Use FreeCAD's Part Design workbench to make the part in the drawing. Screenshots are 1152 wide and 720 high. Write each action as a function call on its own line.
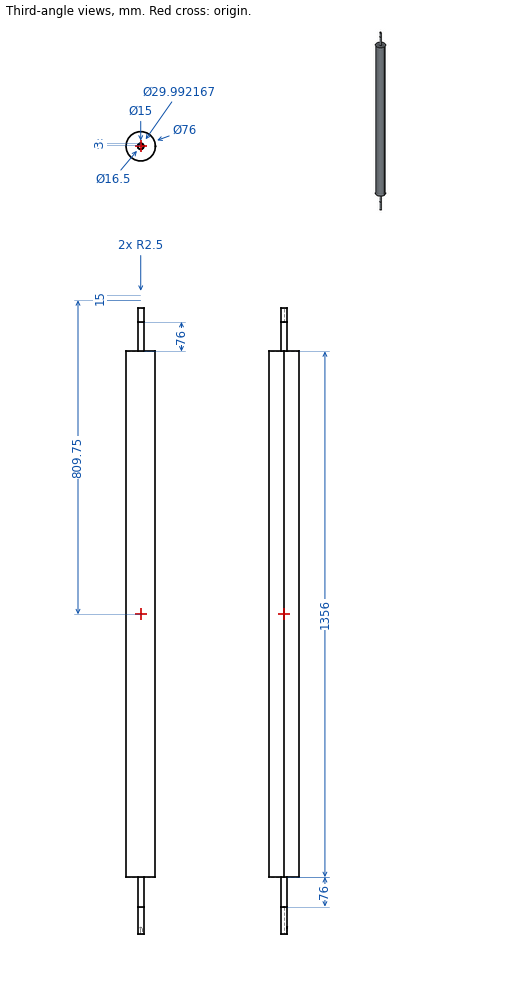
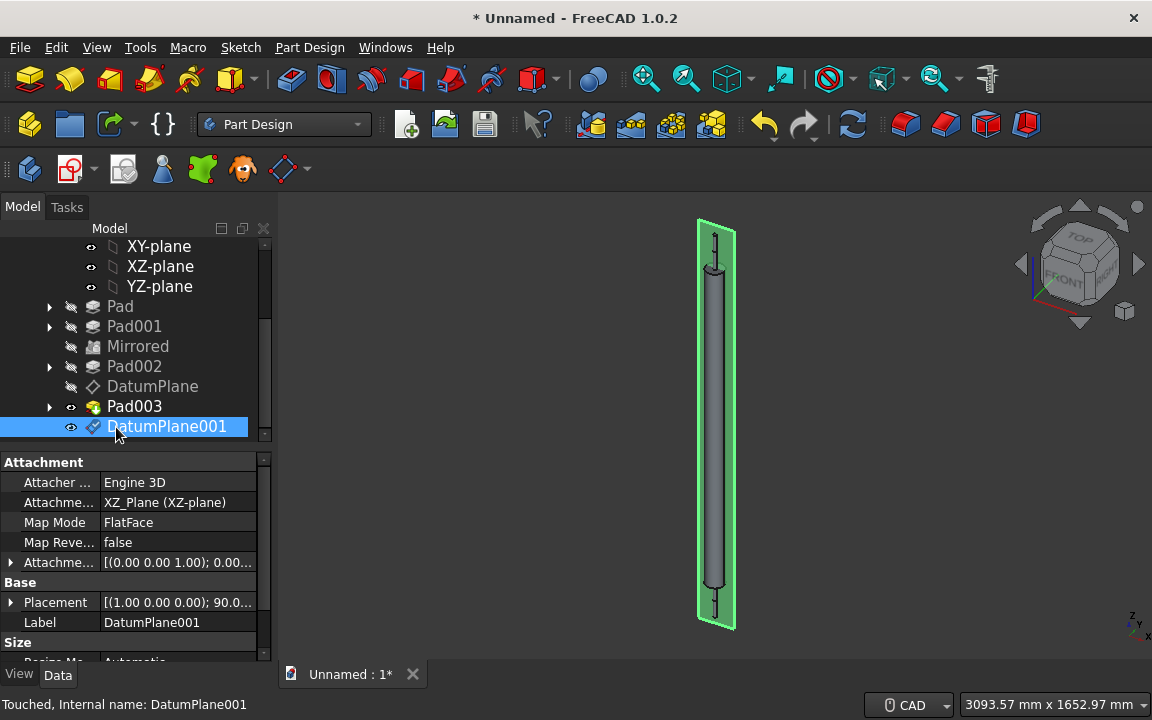
click(70, 170)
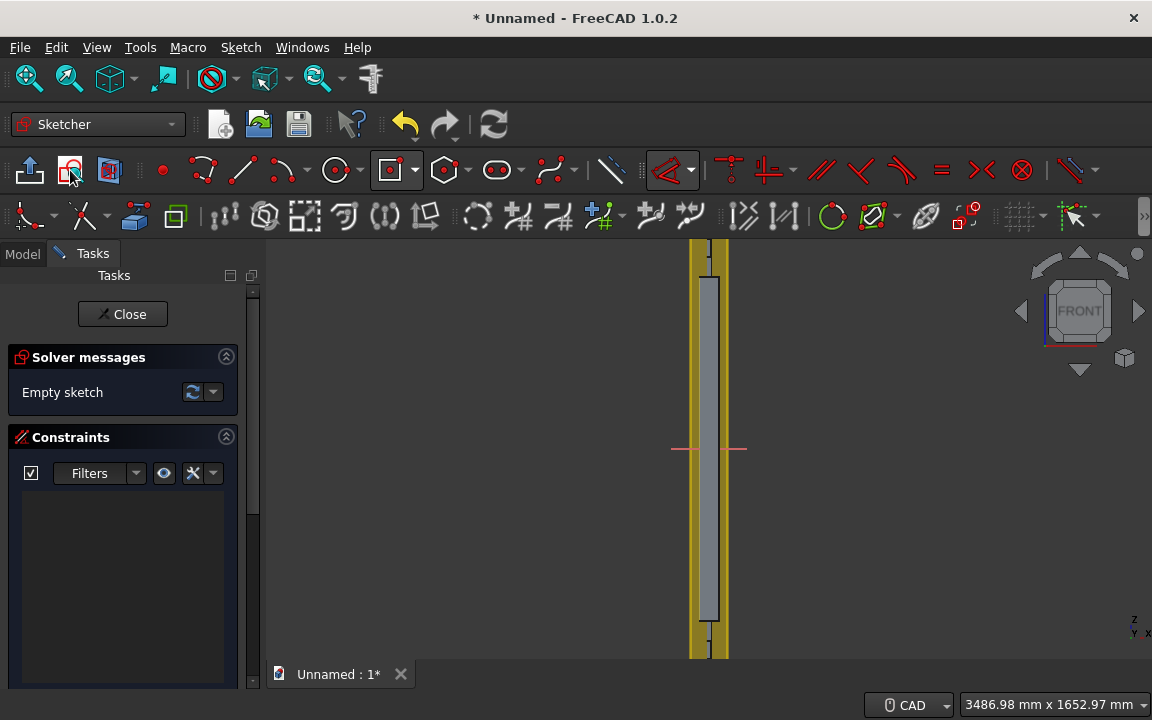
click(110, 170)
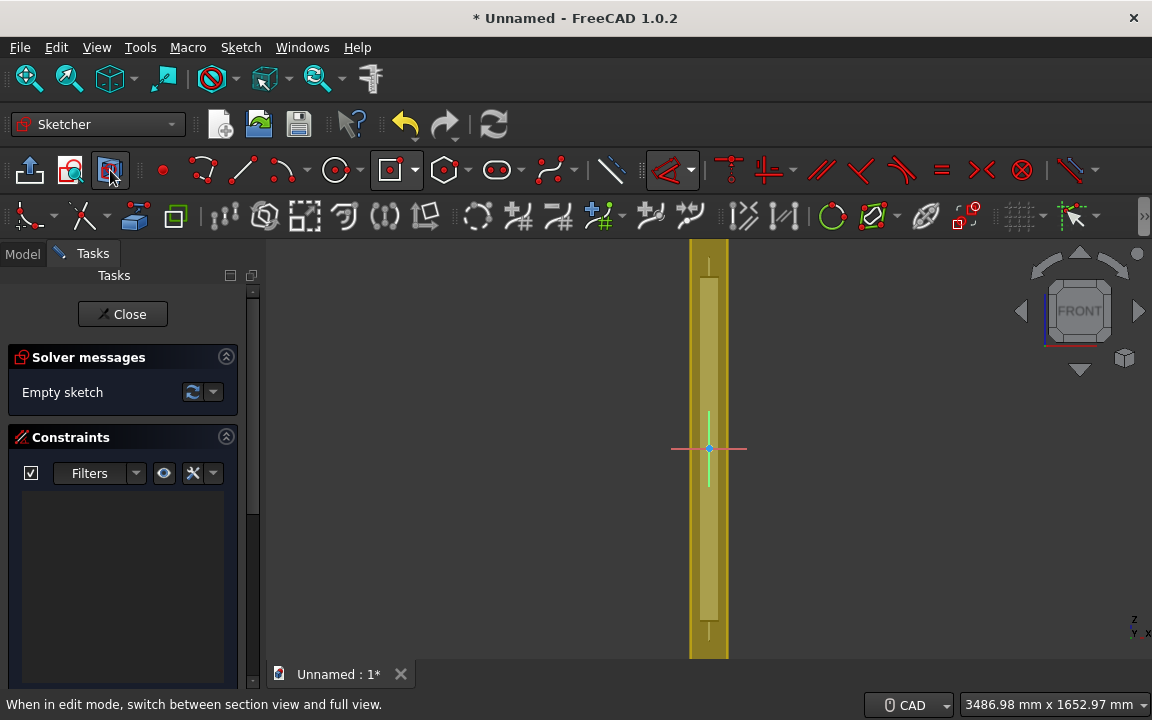
scroll(640, 449, down, 5)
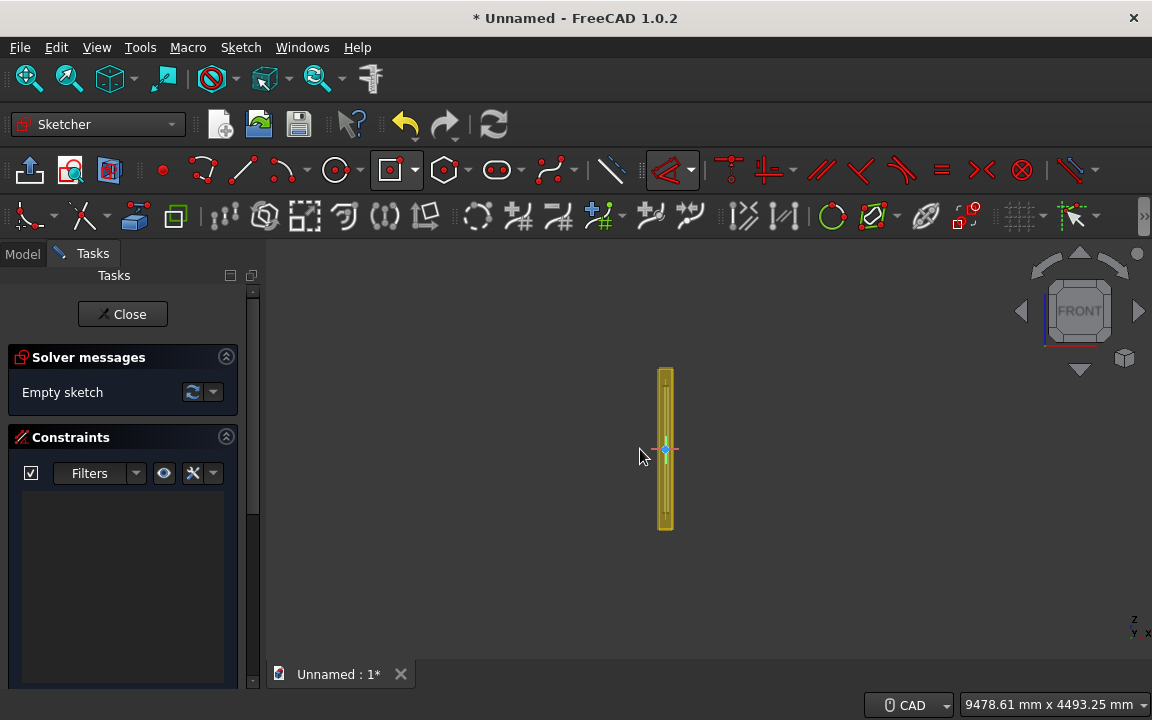
scroll(667, 369, up, 15)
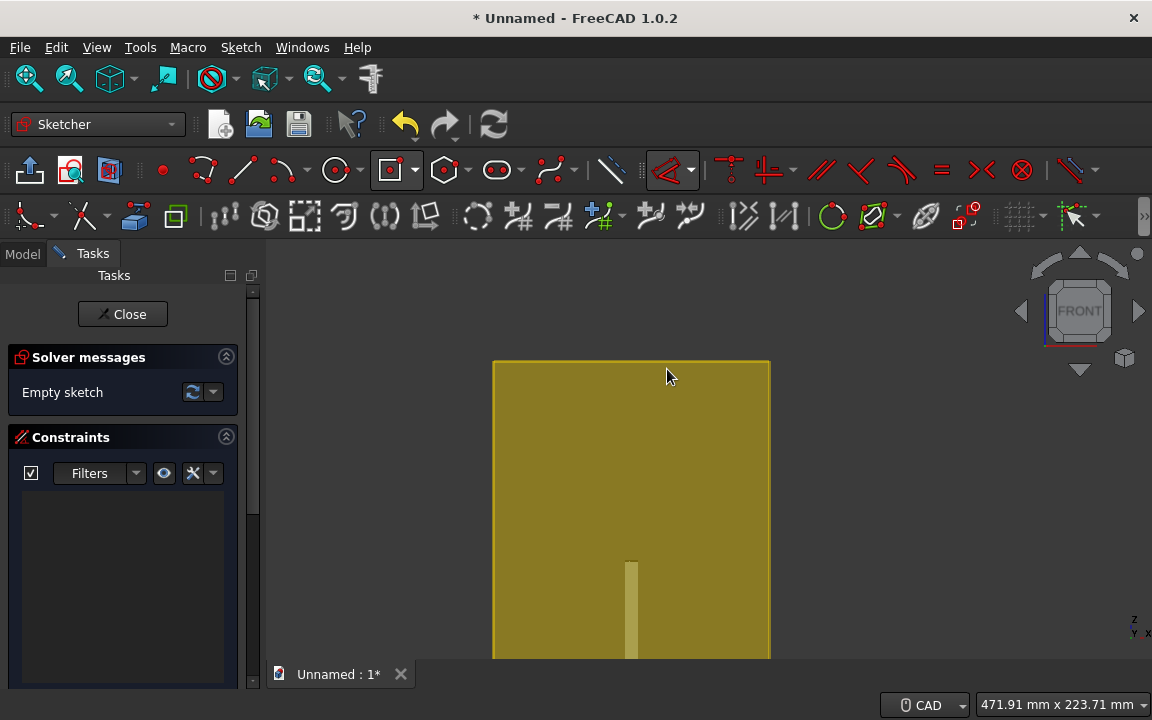
scroll(630, 441, up, 10)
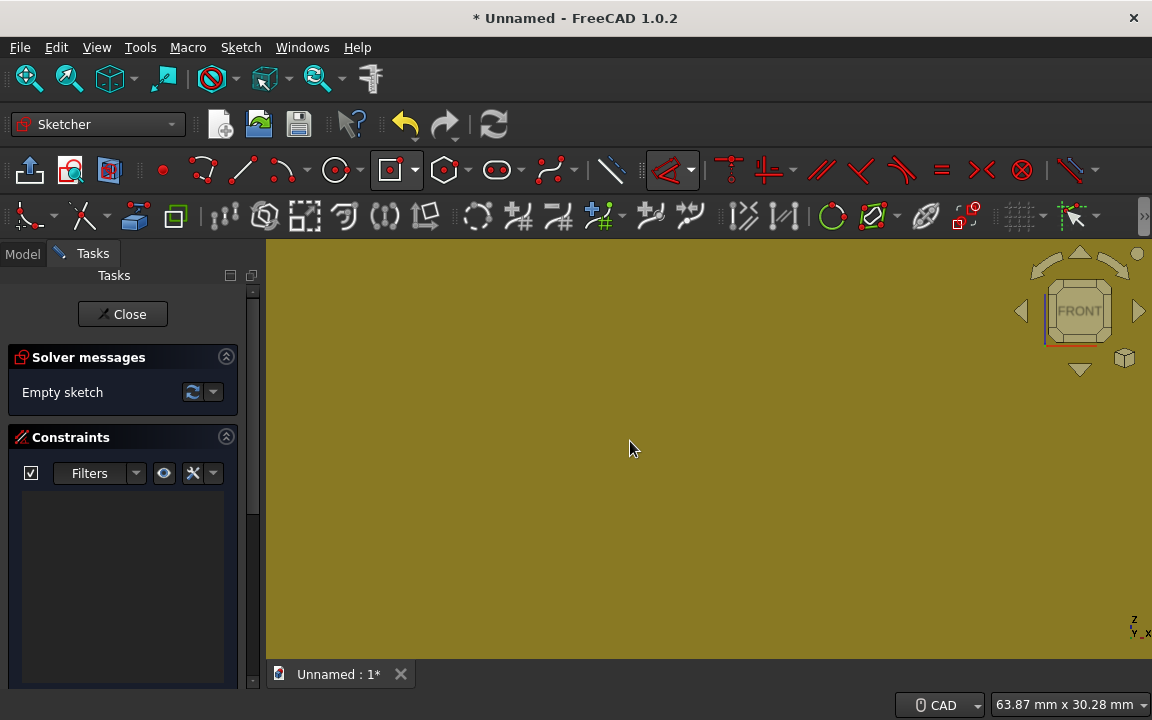
click(498, 170)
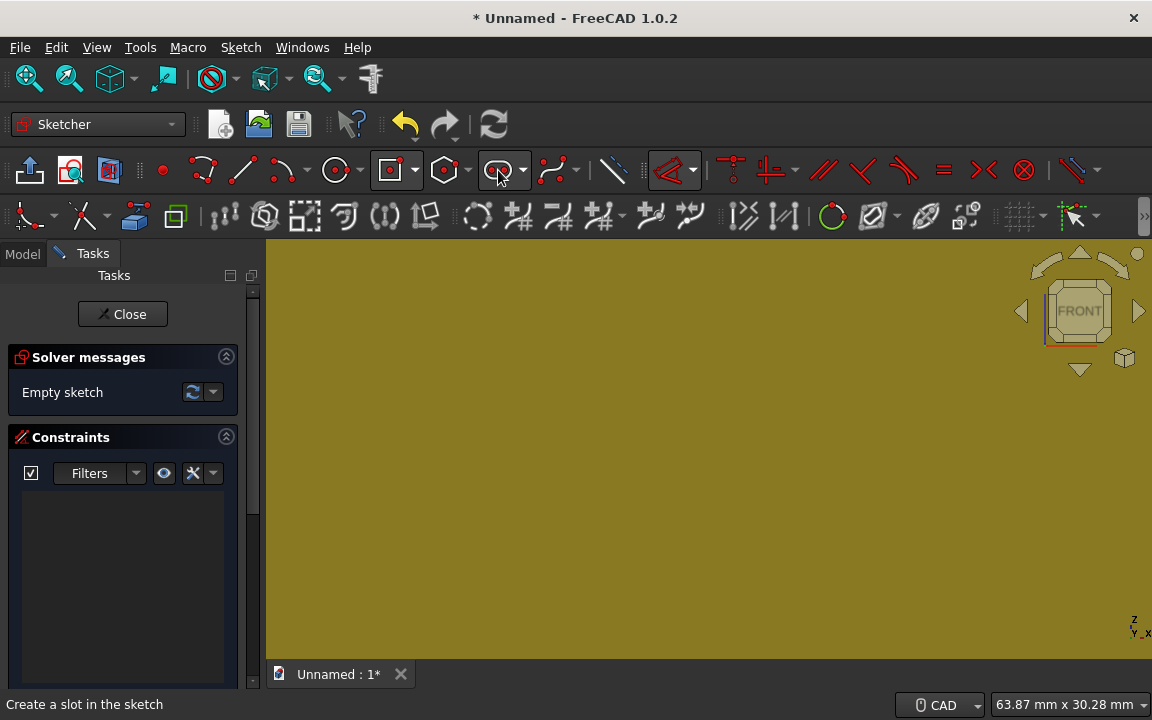
click(637, 549)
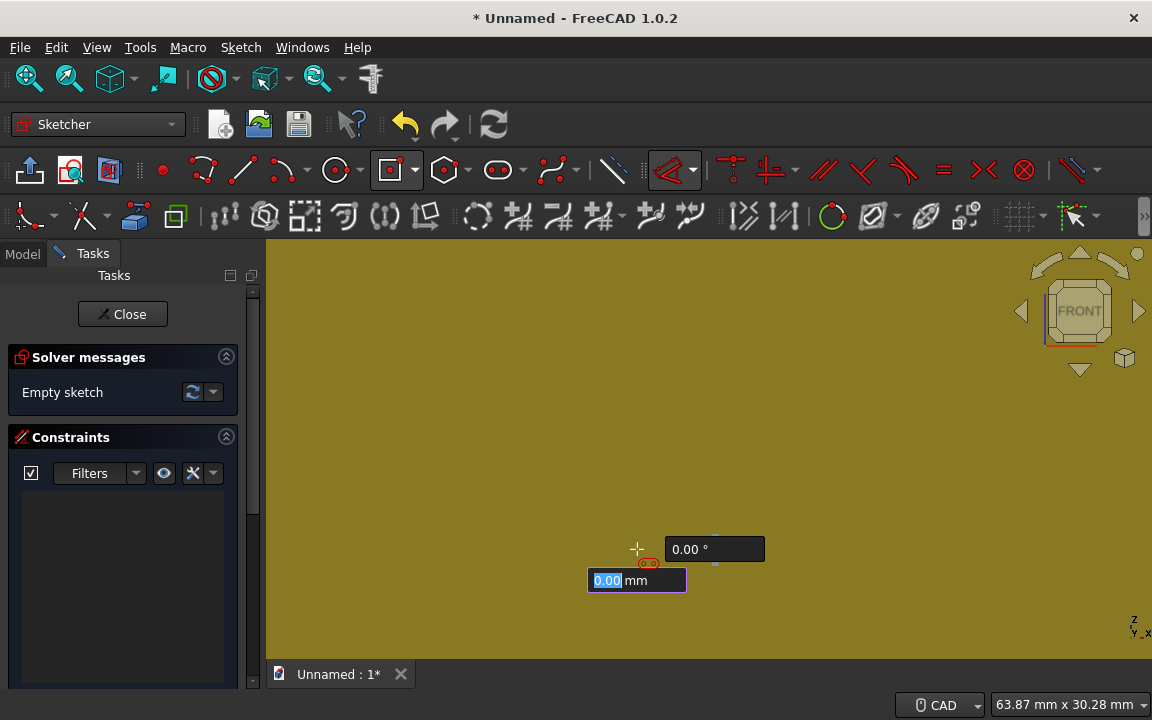
click(646, 341)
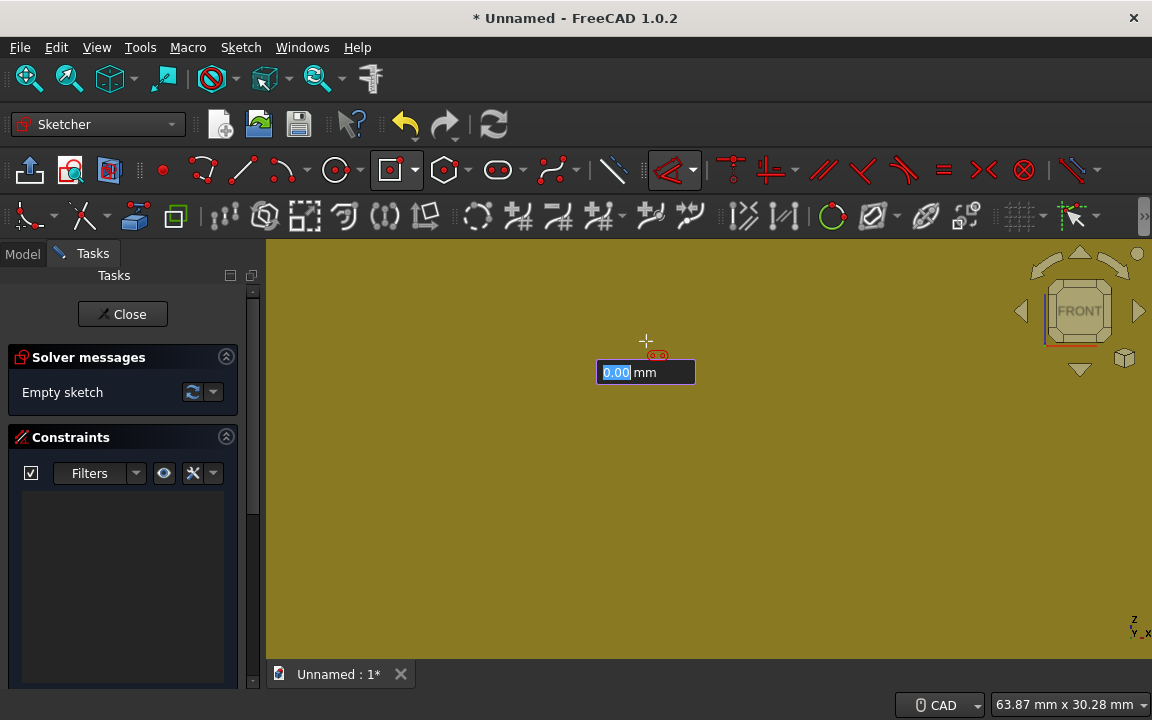
click(602, 445)
key(Escape)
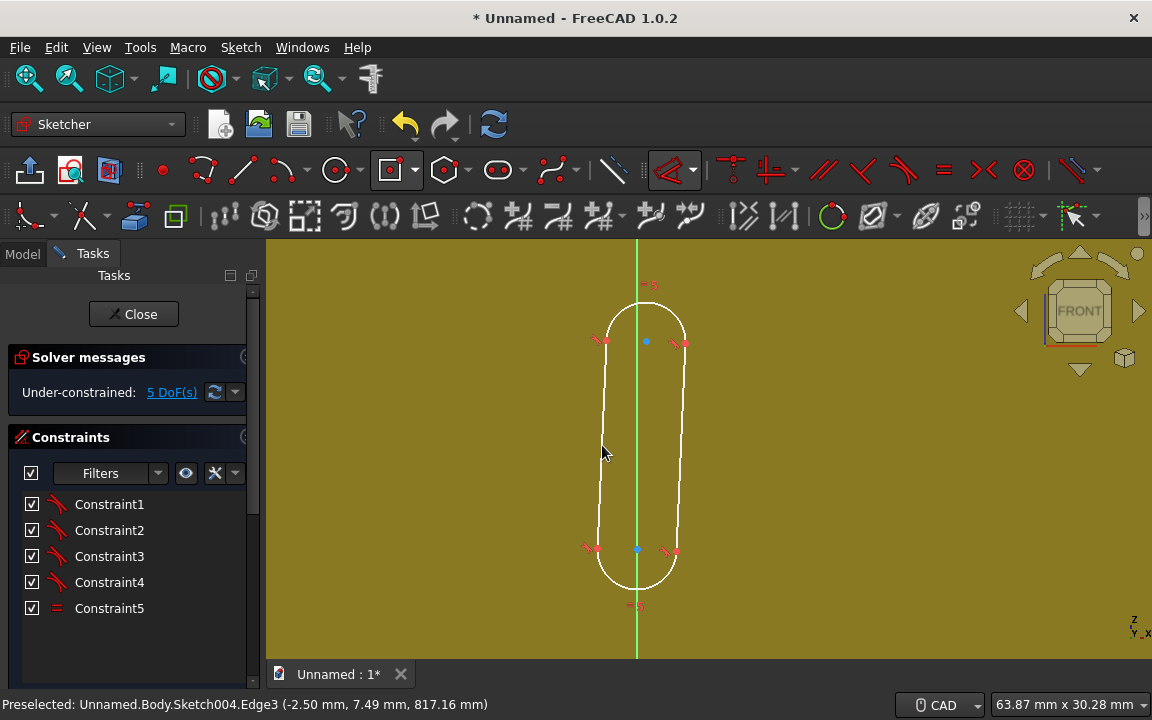
click(600, 486)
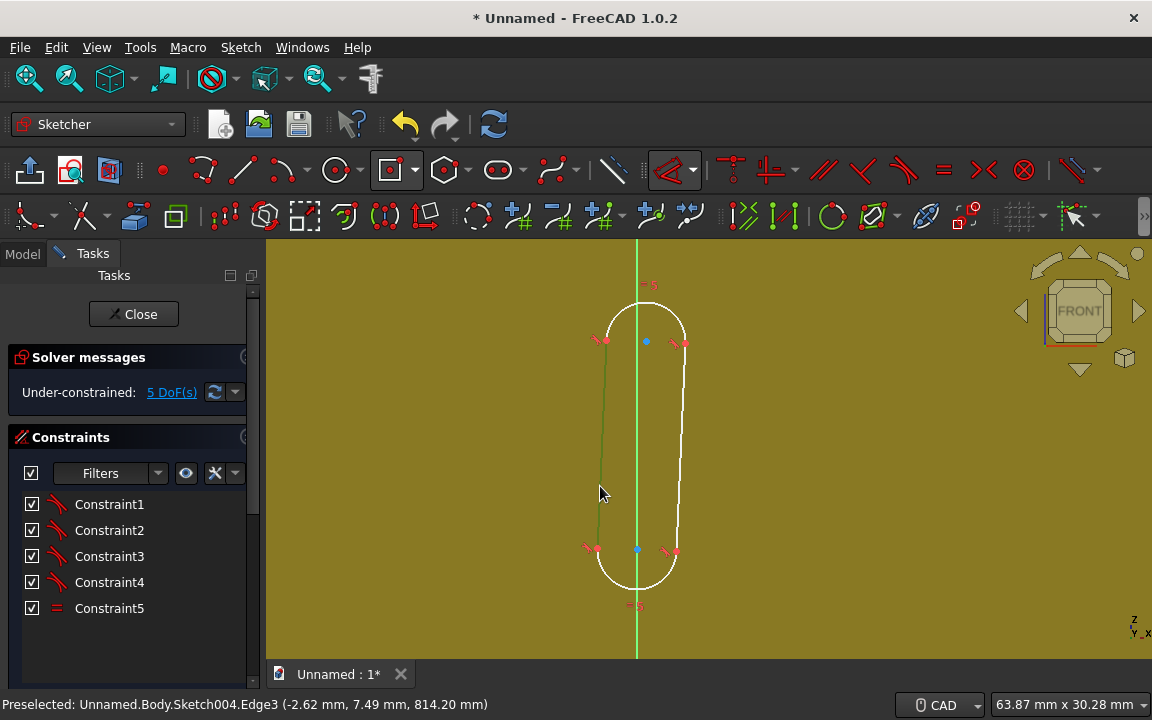
key(v)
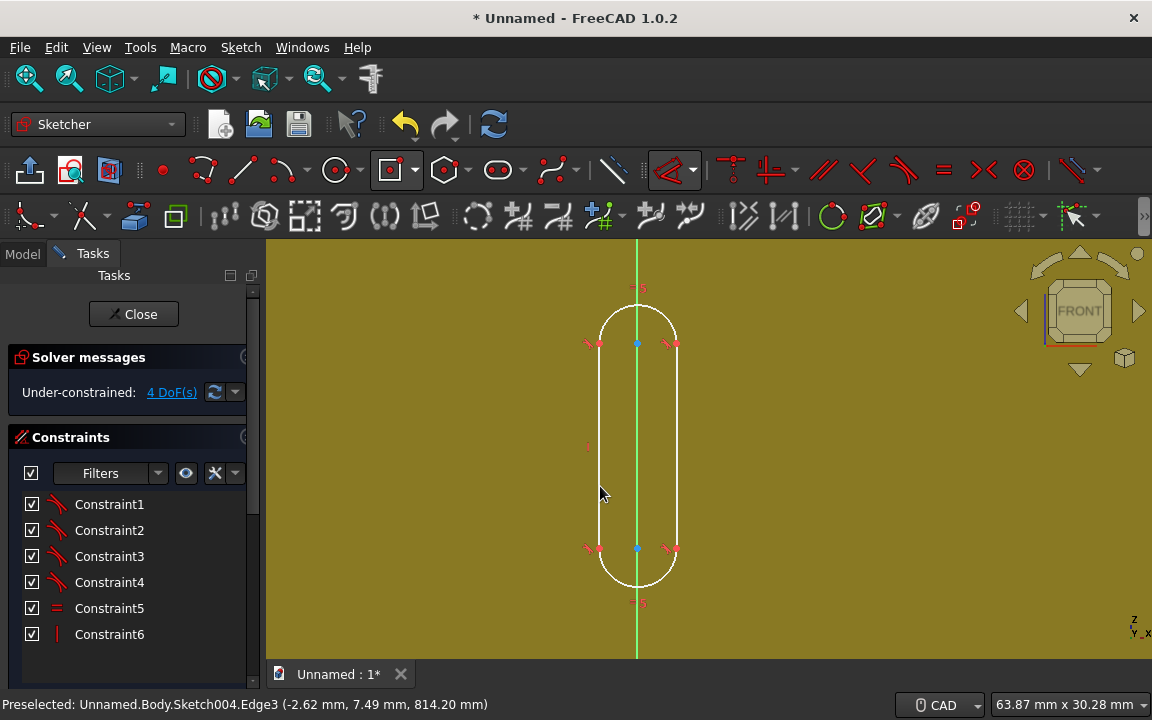
click(638, 548)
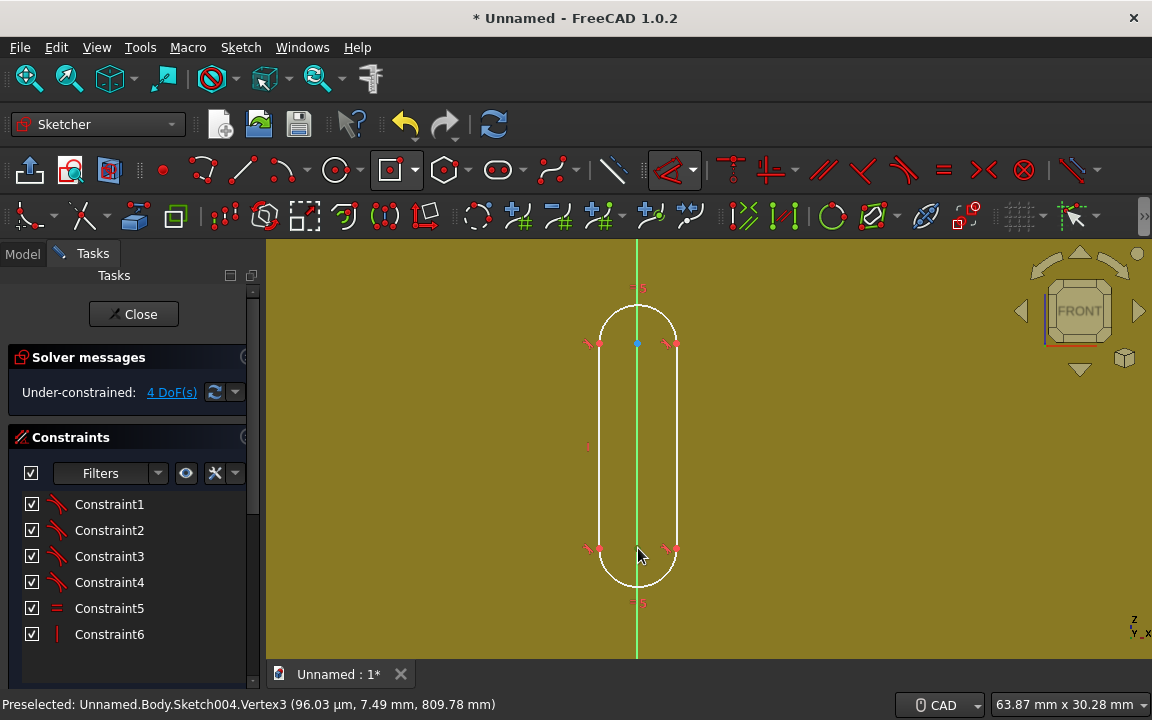
click(637, 553)